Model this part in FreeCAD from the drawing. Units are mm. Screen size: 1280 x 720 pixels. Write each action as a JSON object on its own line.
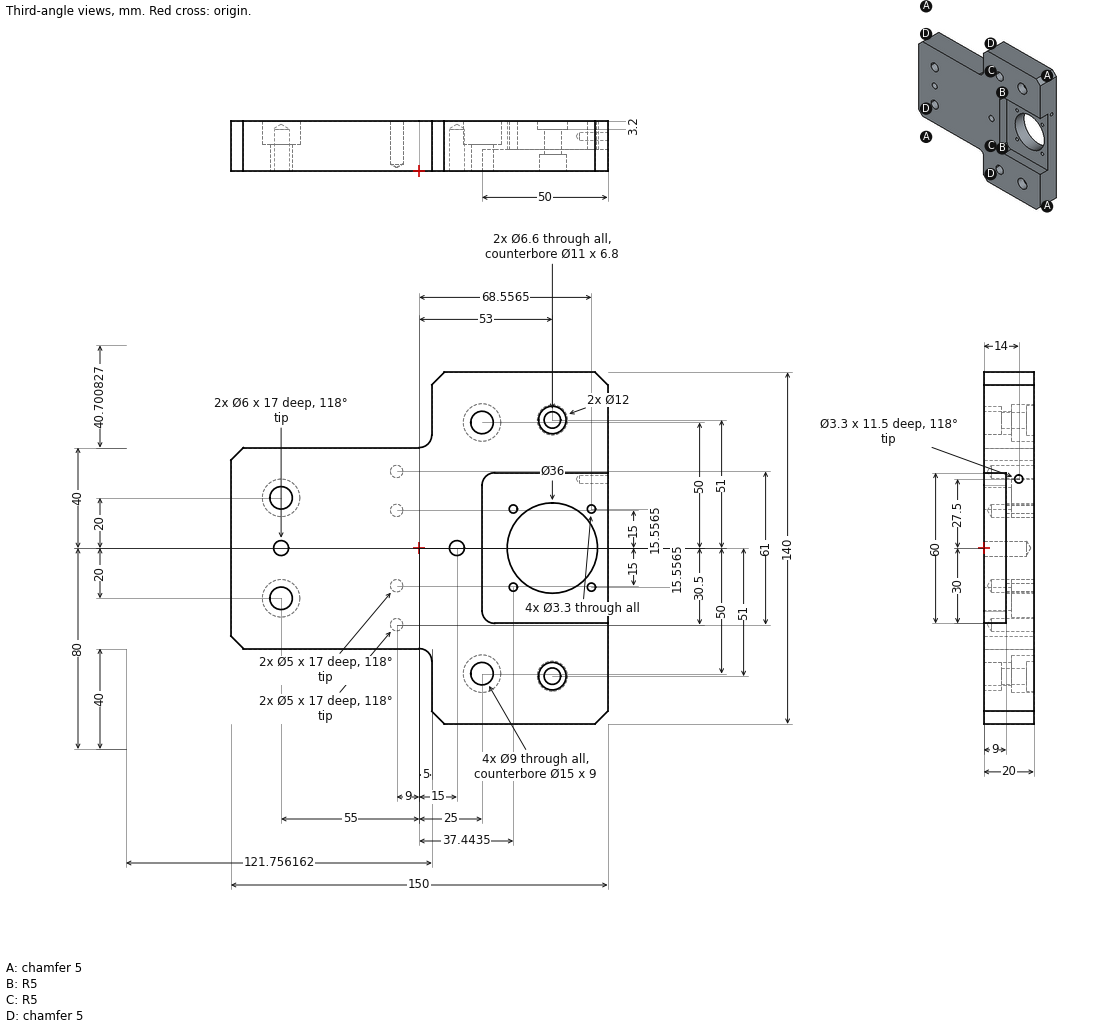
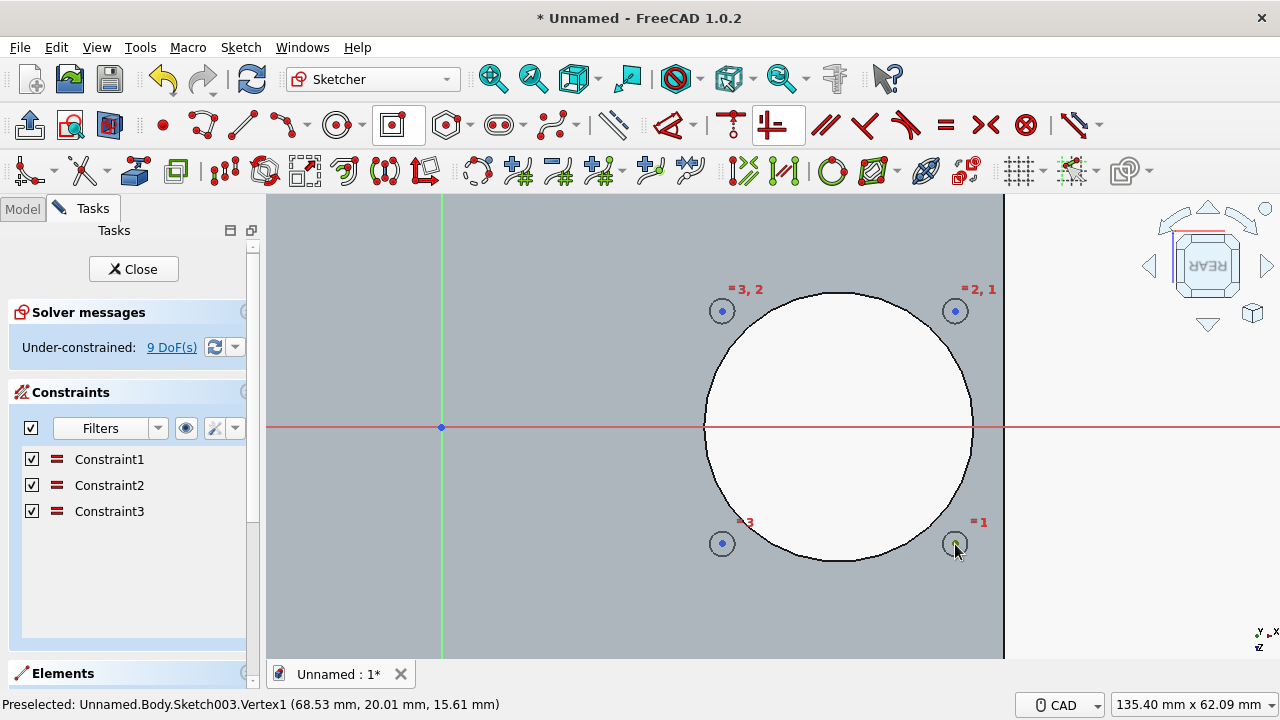
{"action": "left_click", "coordinate": [955, 311]}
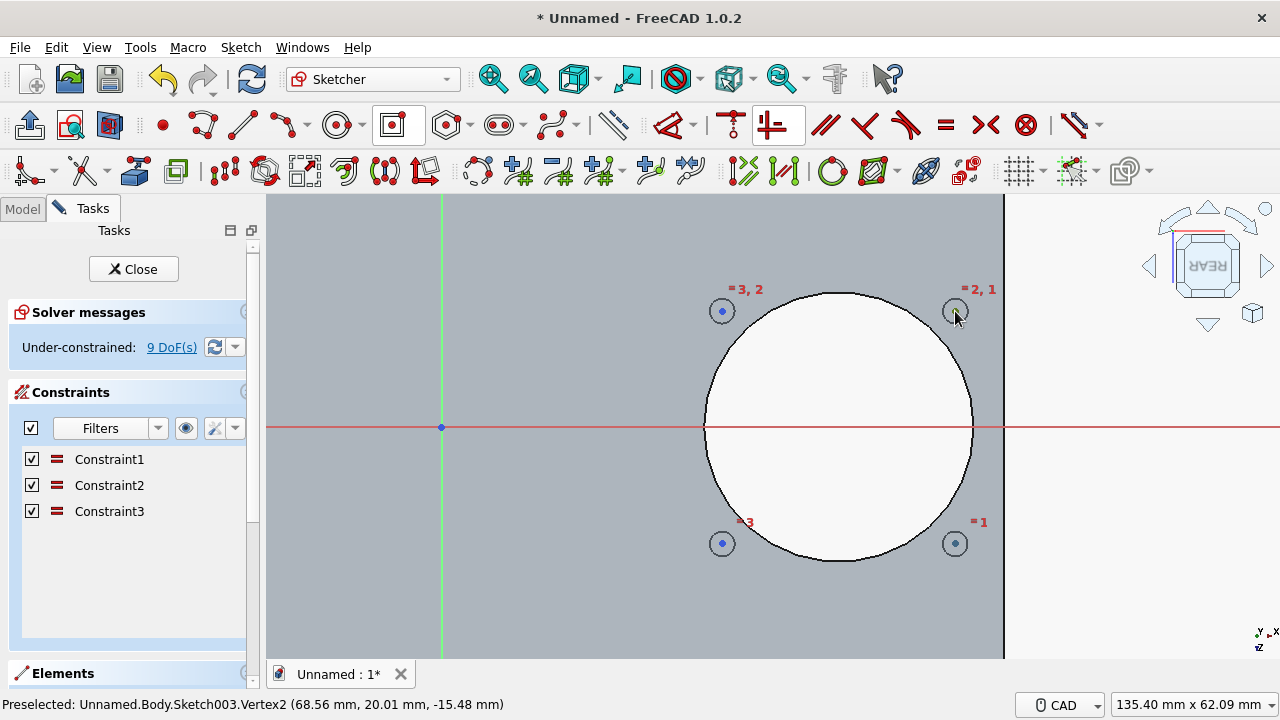
{"action": "left_click", "coordinate": [800, 126]}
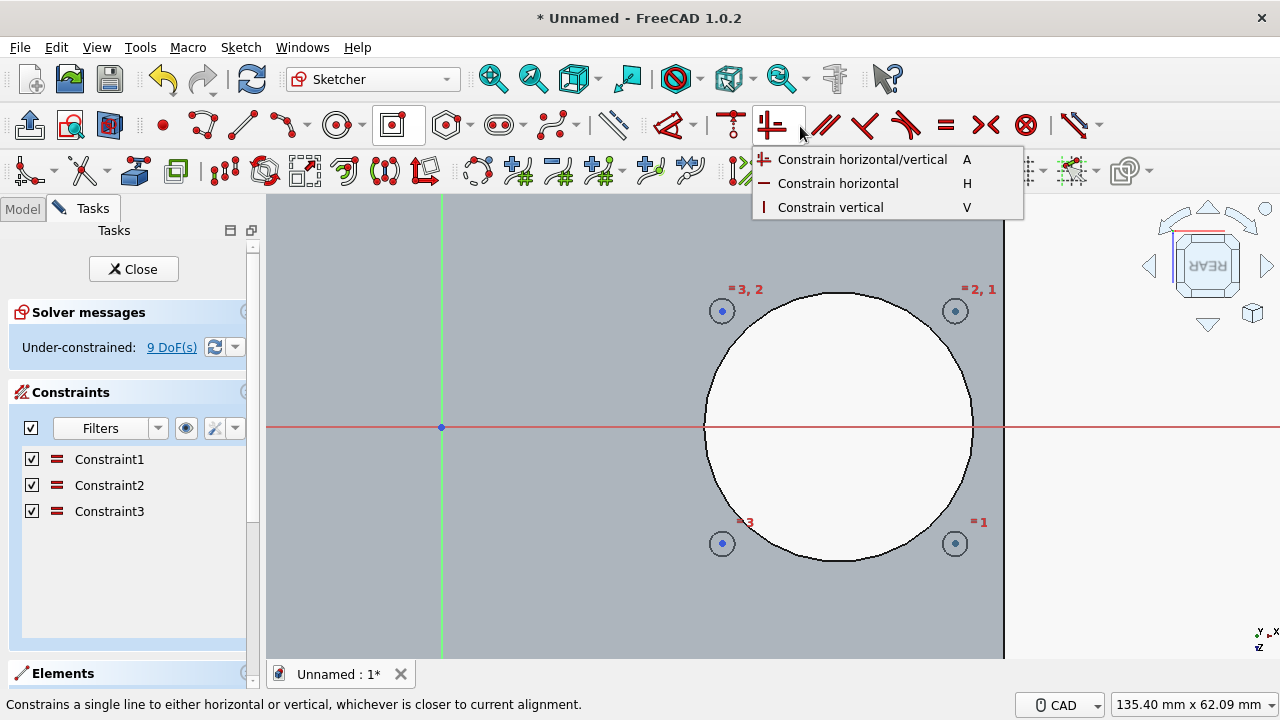
{"action": "left_click", "coordinate": [888, 207]}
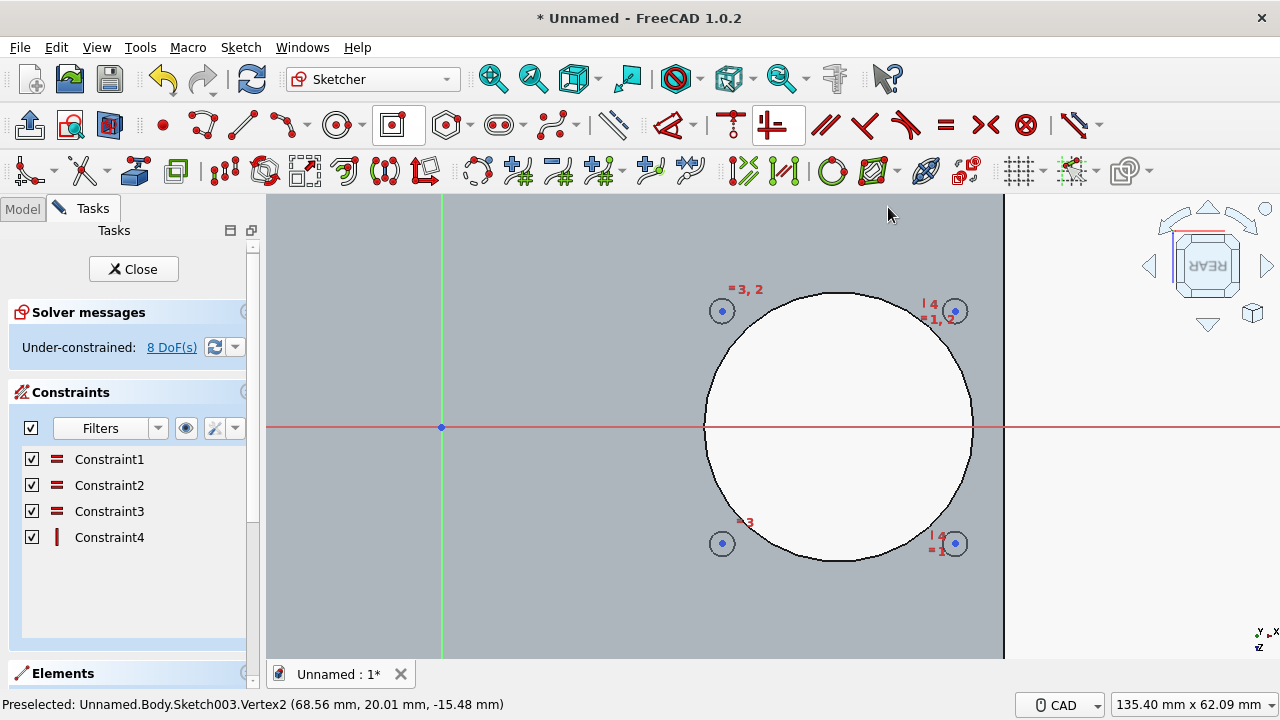
{"action": "left_click", "coordinate": [955, 311]}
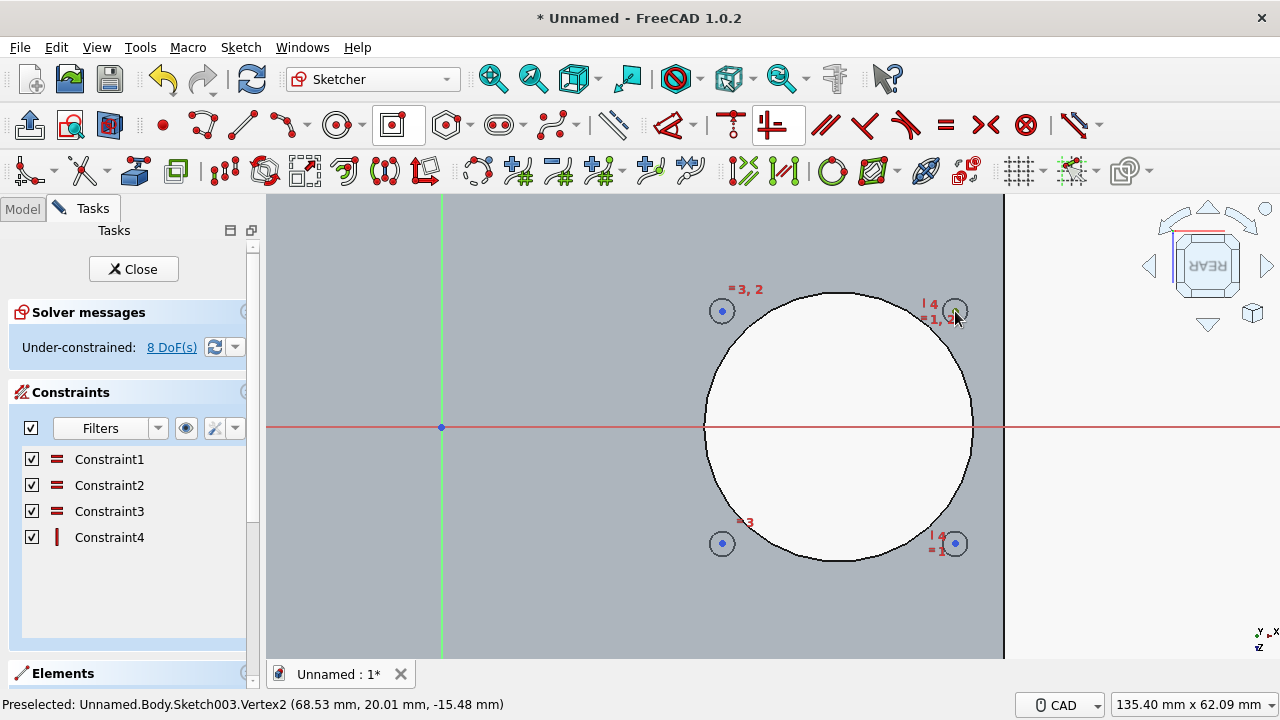
{"action": "left_click", "coordinate": [722, 311]}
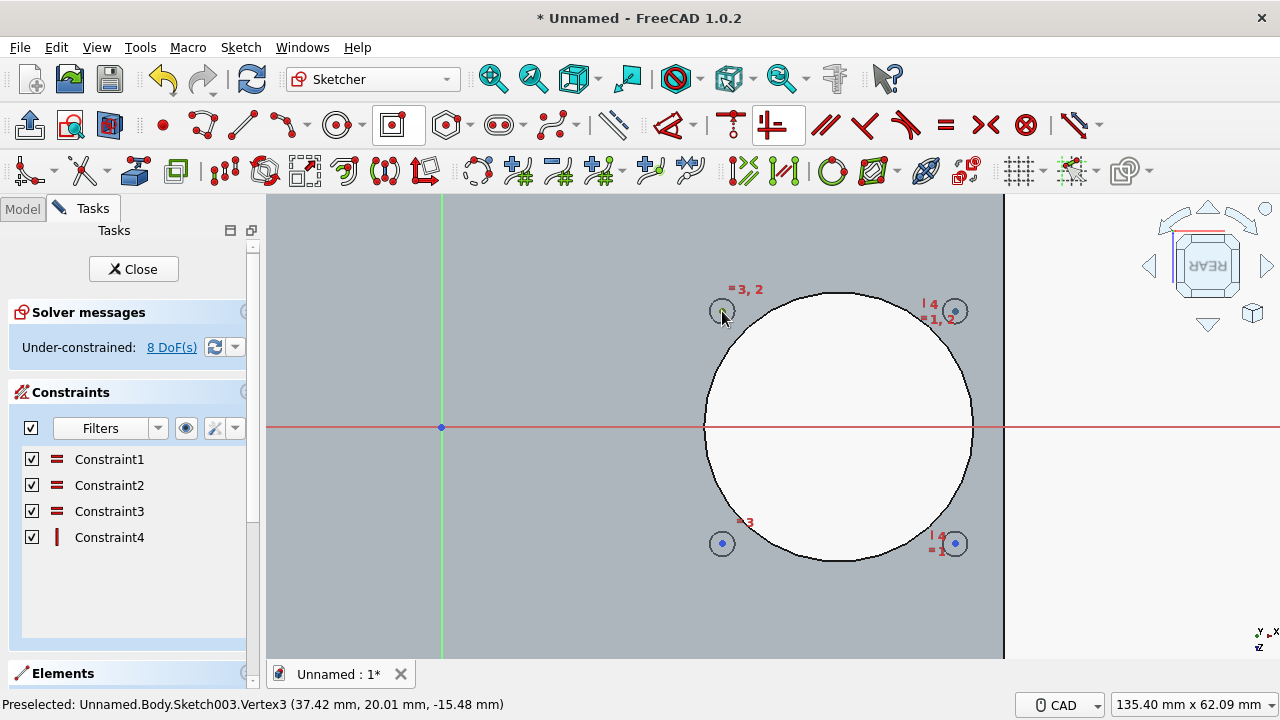
{"action": "left_click", "coordinate": [800, 126]}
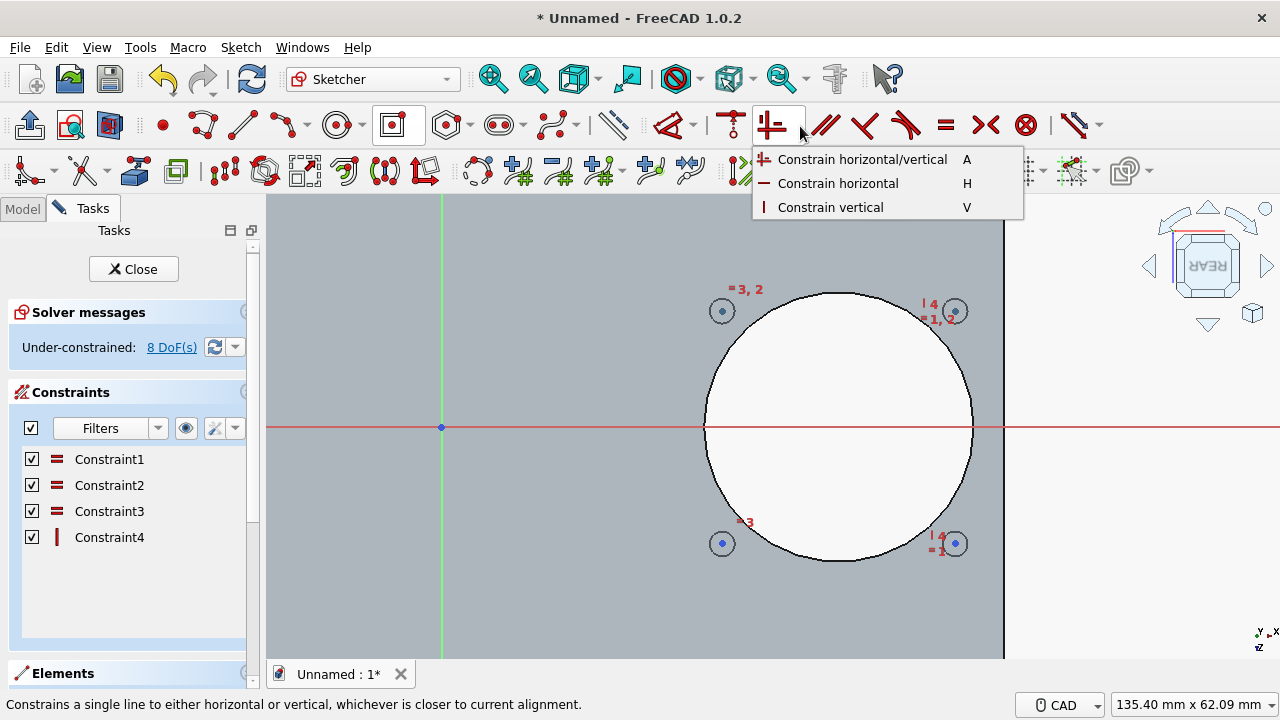
{"action": "left_click", "coordinate": [888, 183]}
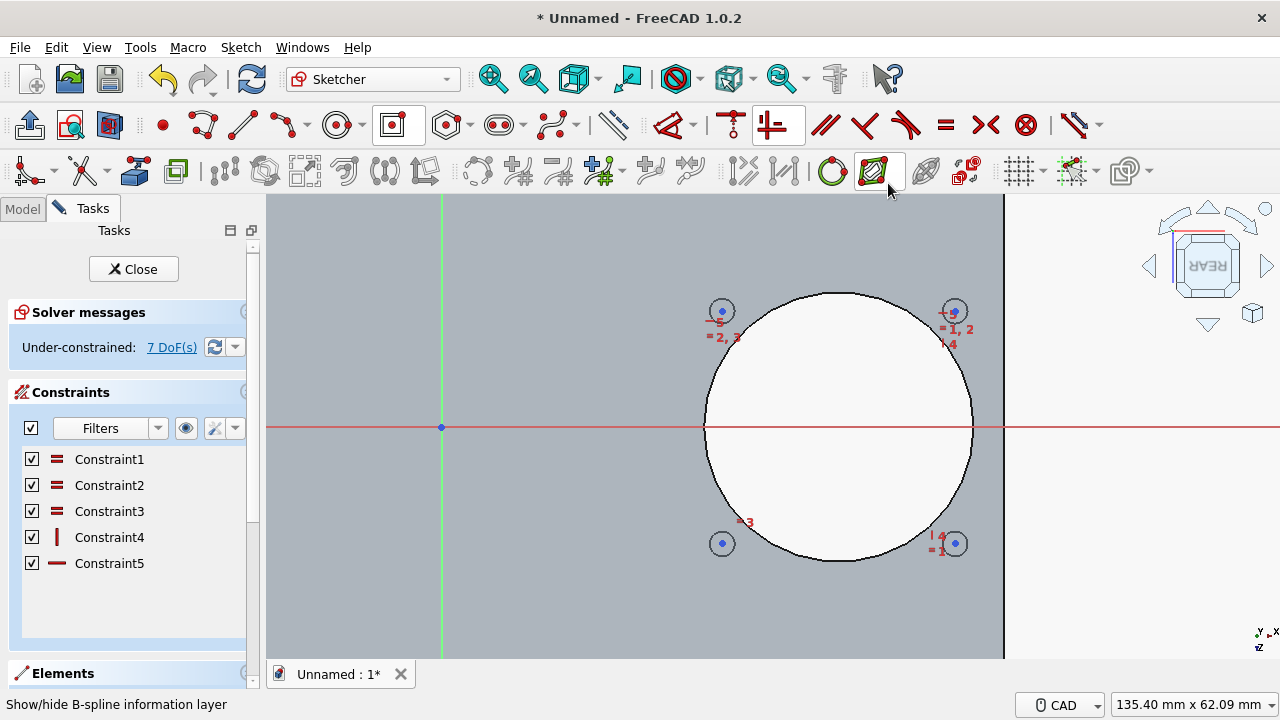
{"action": "left_click", "coordinate": [722, 311]}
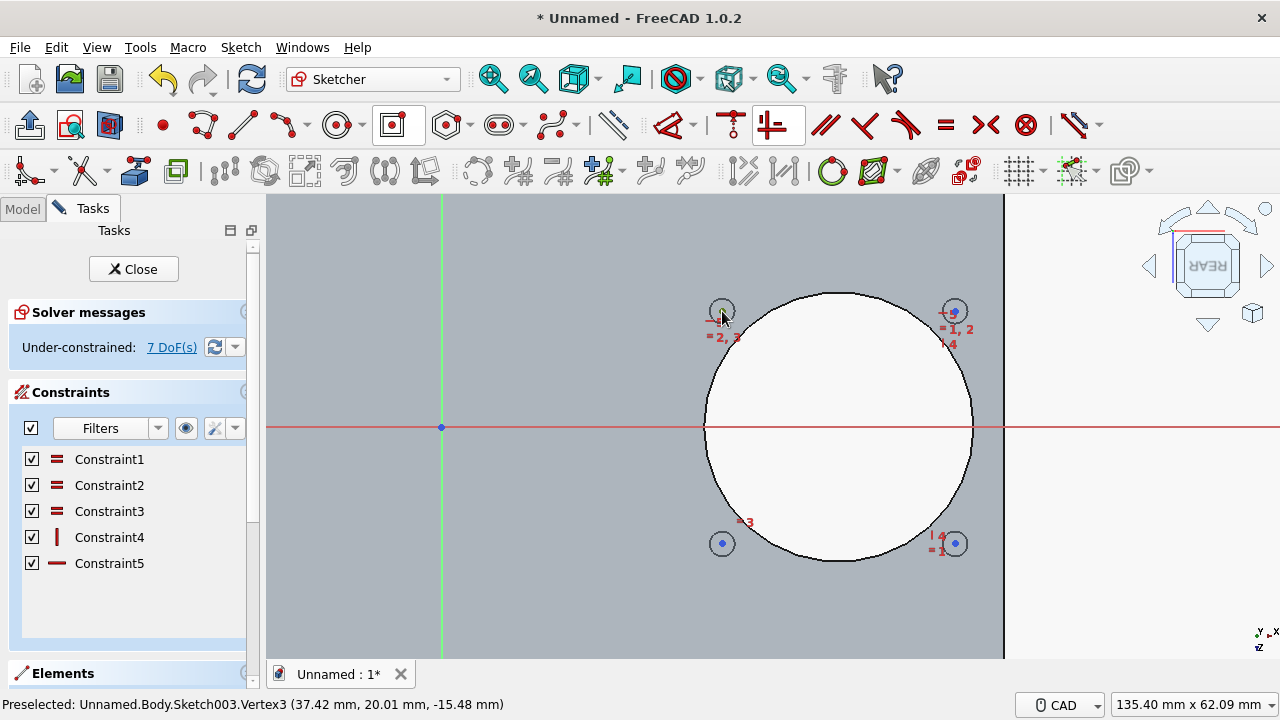
{"action": "left_click", "coordinate": [722, 544]}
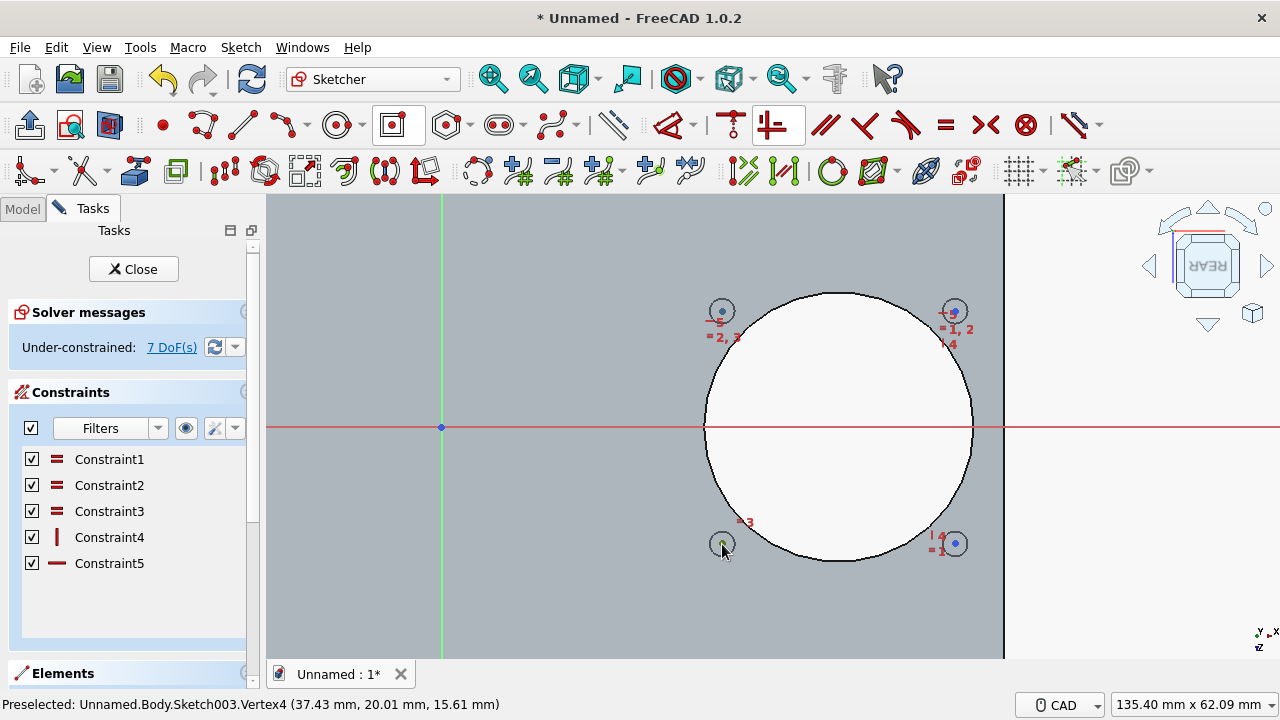
{"action": "key", "text": "v"}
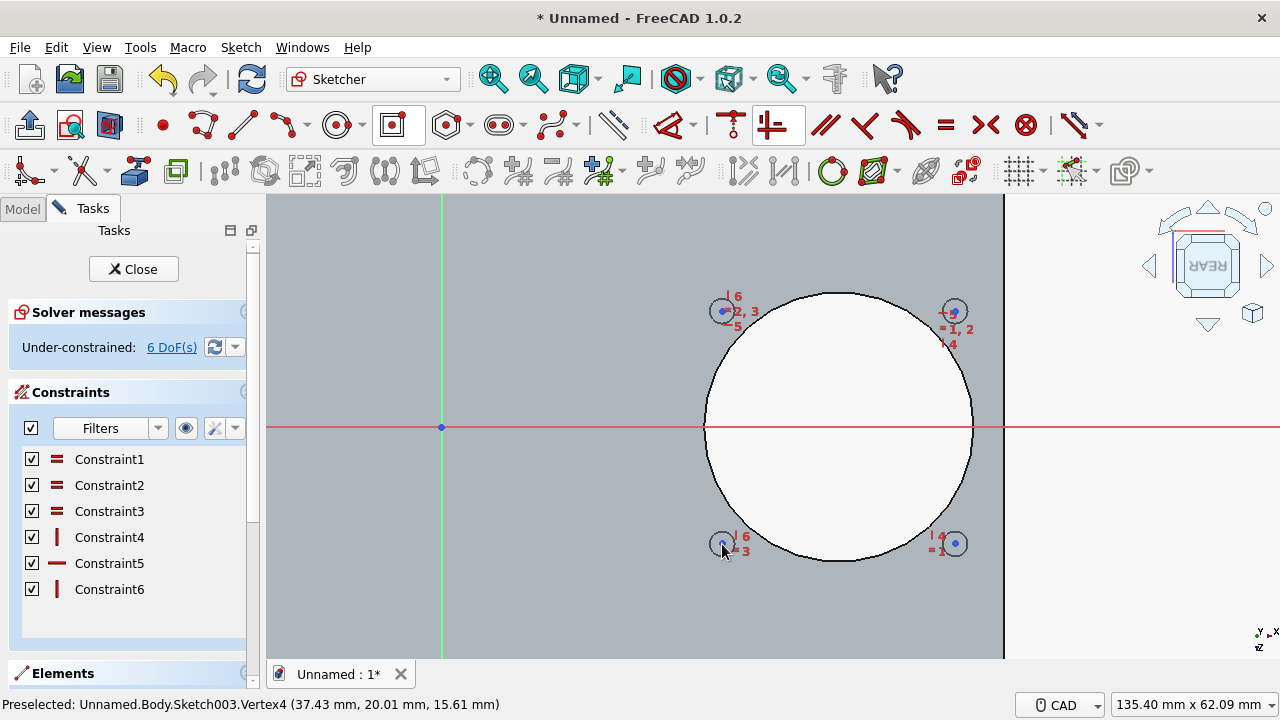
{"action": "left_click", "coordinate": [955, 544]}